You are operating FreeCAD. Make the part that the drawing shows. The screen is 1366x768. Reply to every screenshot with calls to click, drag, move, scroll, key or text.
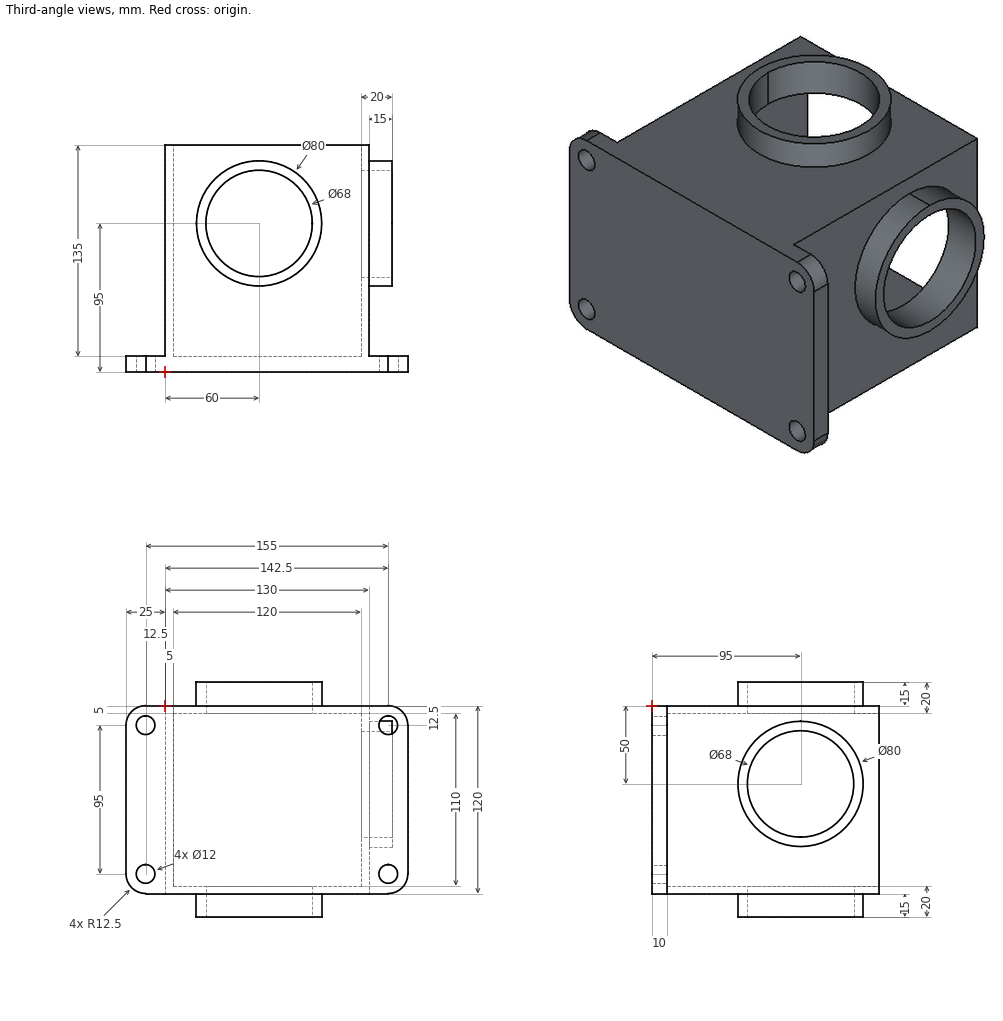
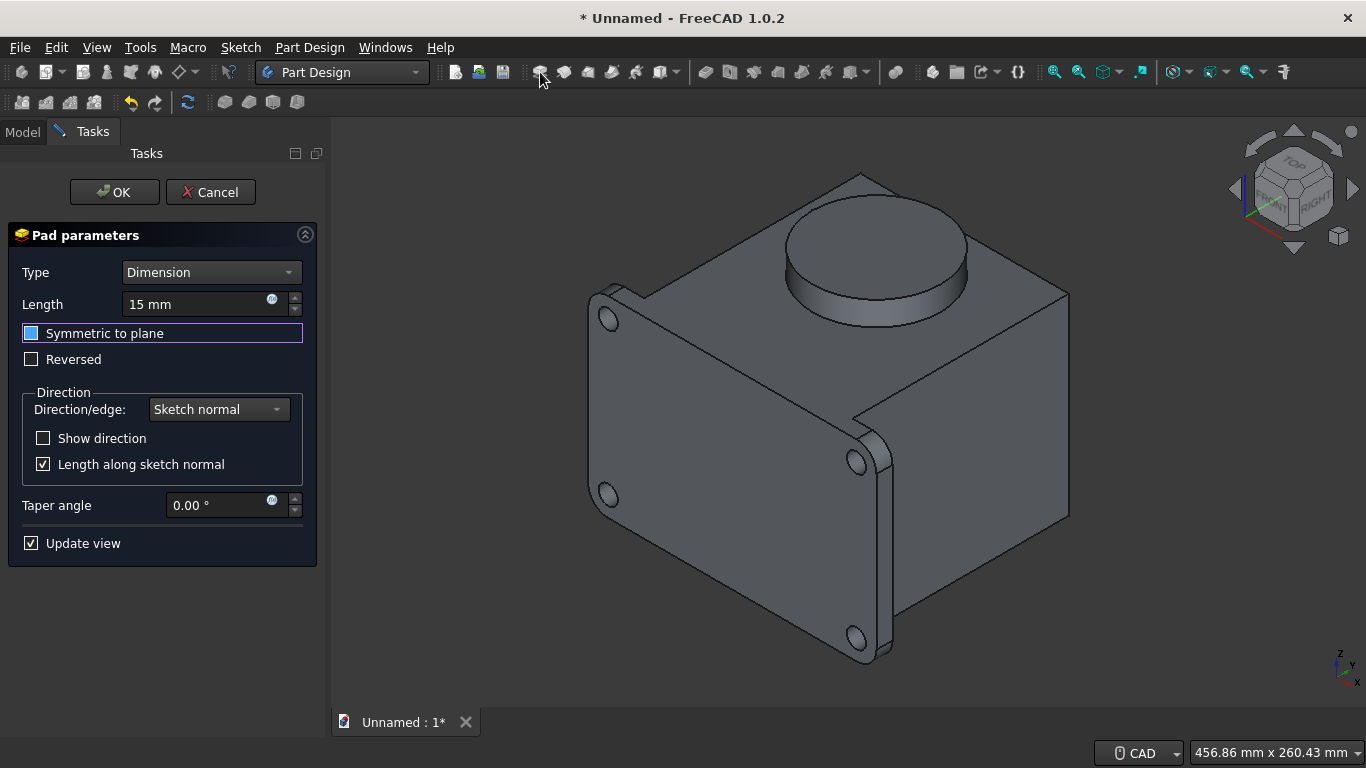
click(115, 192)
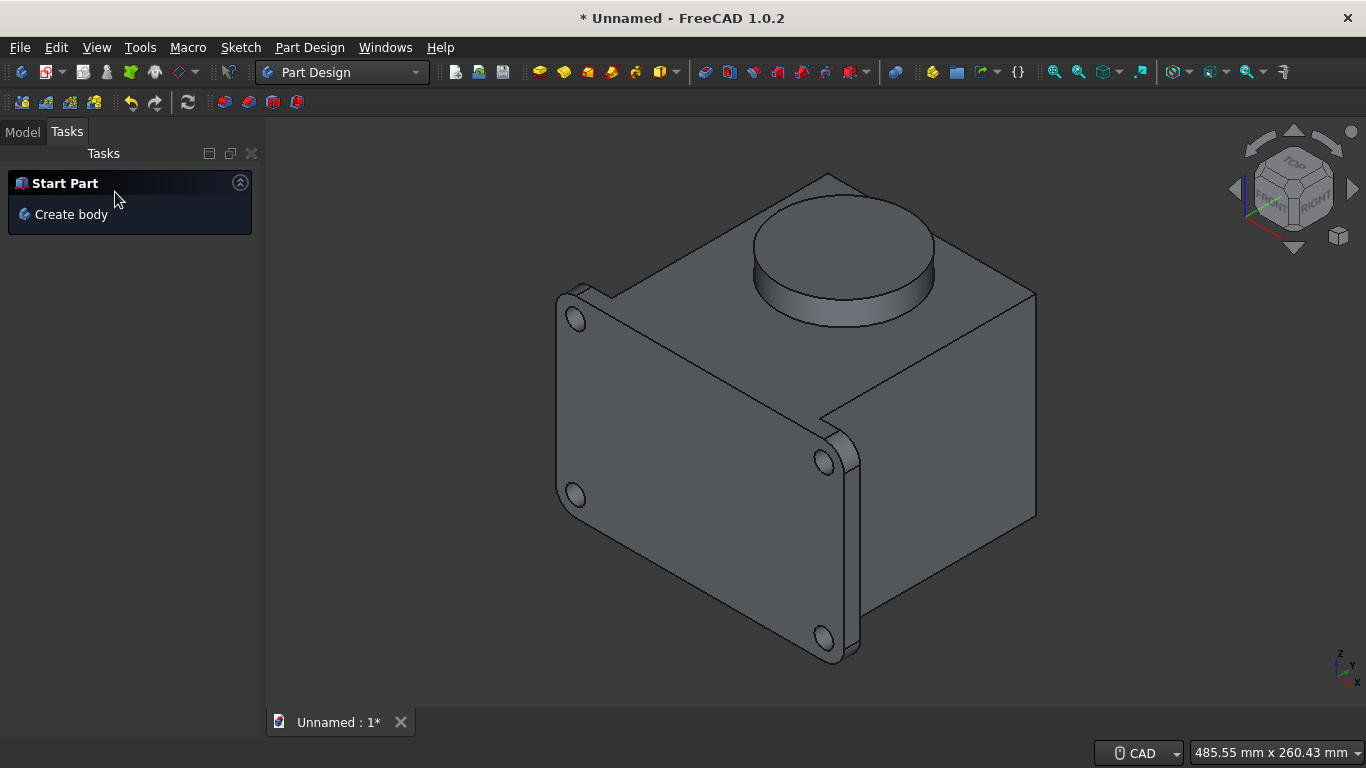
click(844, 246)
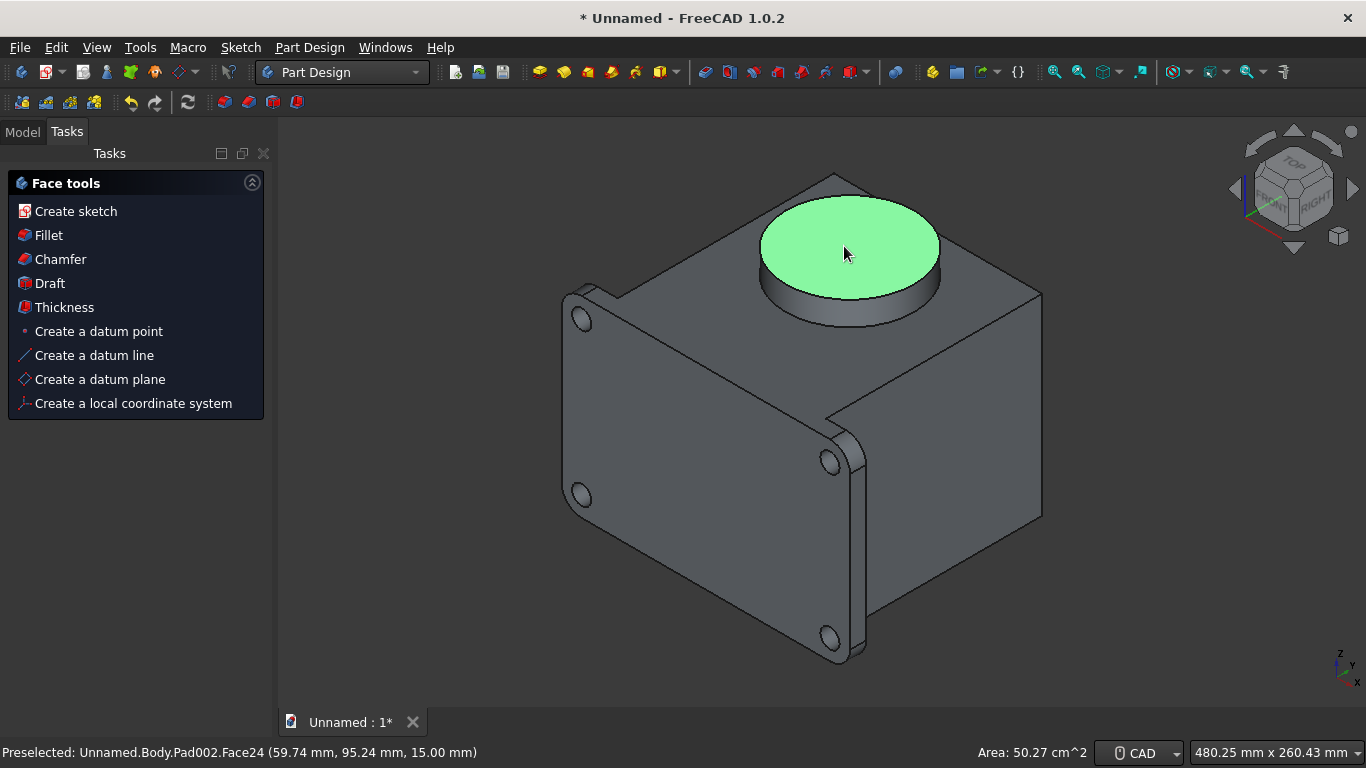
click(46, 72)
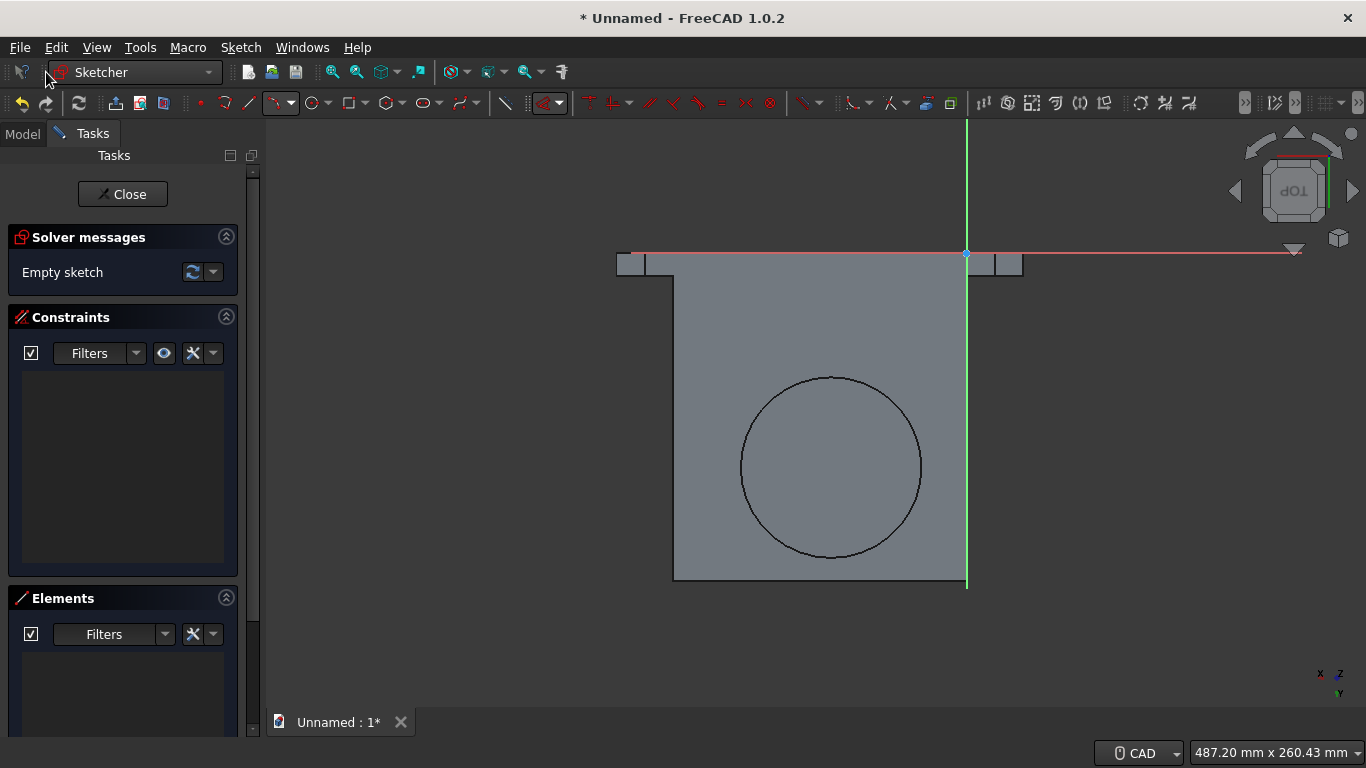
click(312, 104)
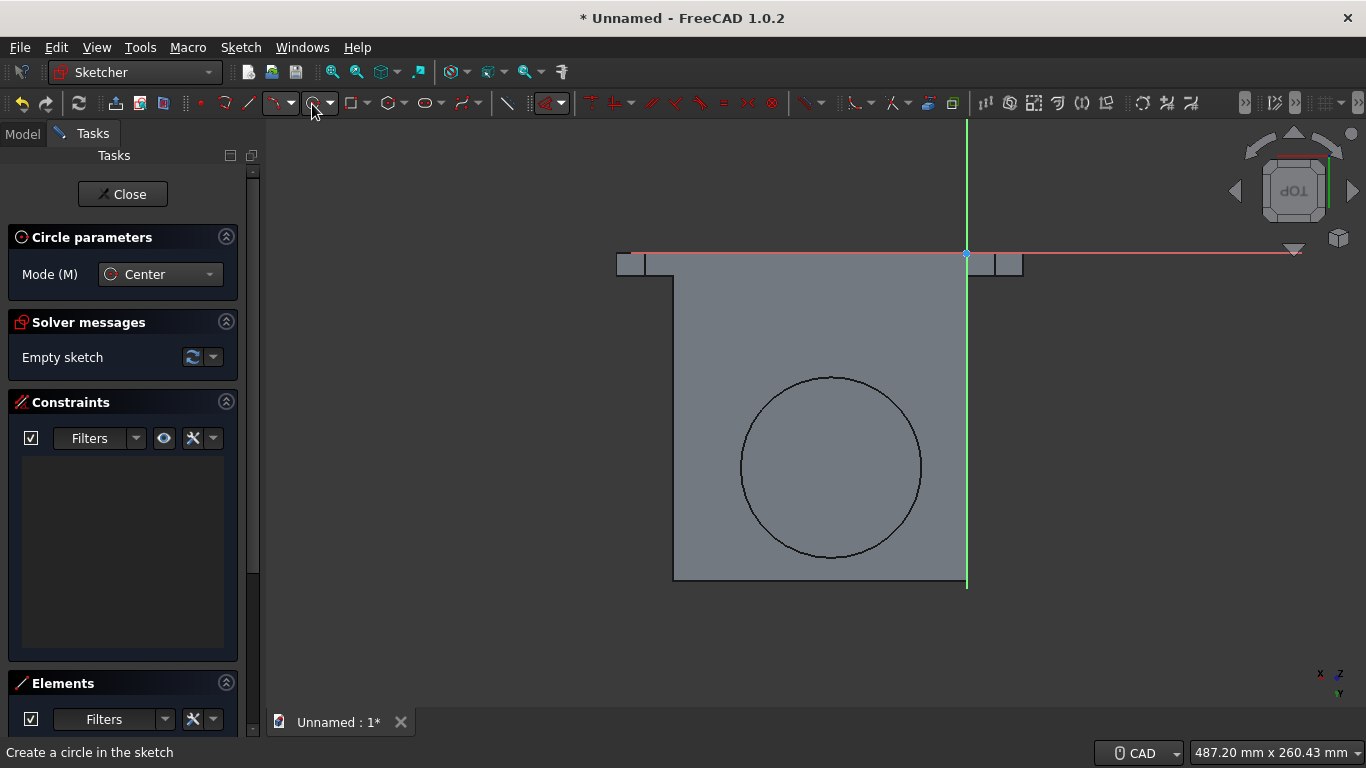
click(831, 468)
move(885, 413)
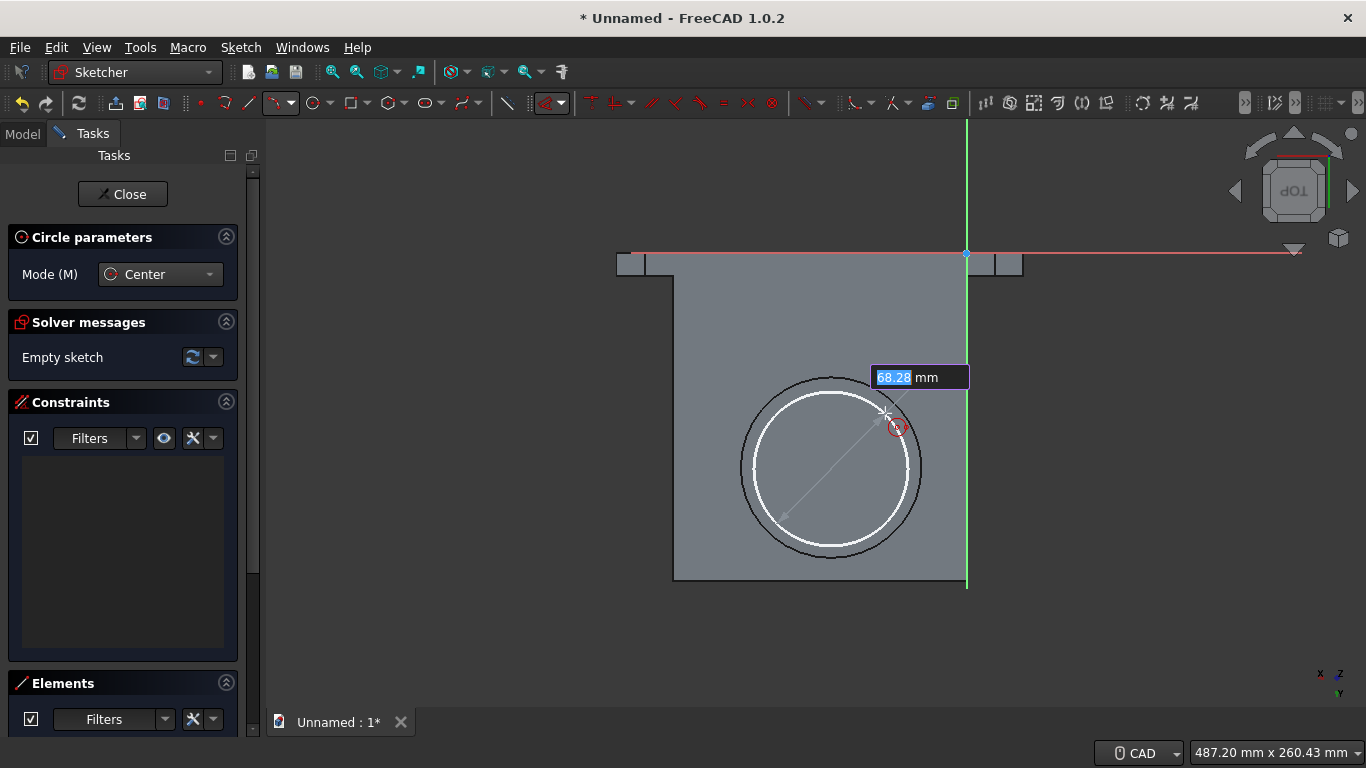
text(68)
key(Return)
key(Escape)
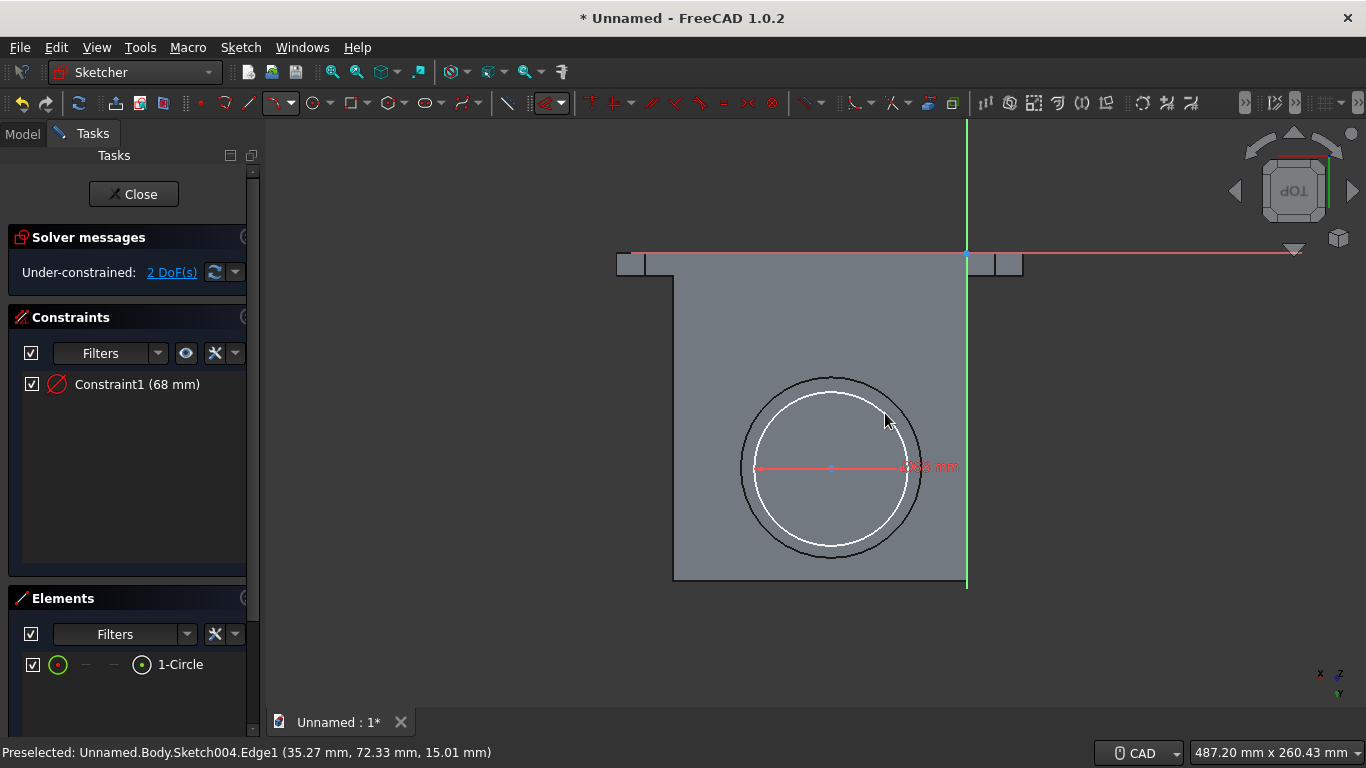
click(831, 469)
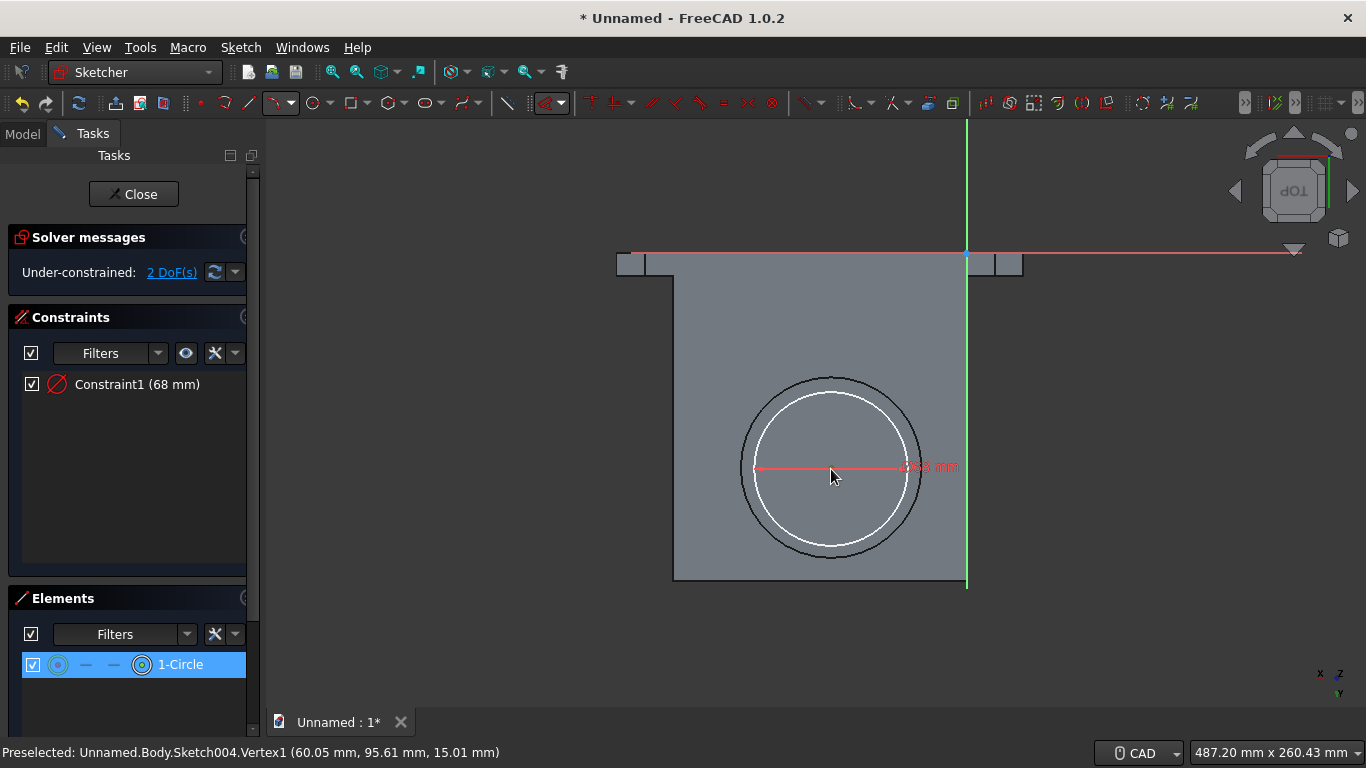
key(l)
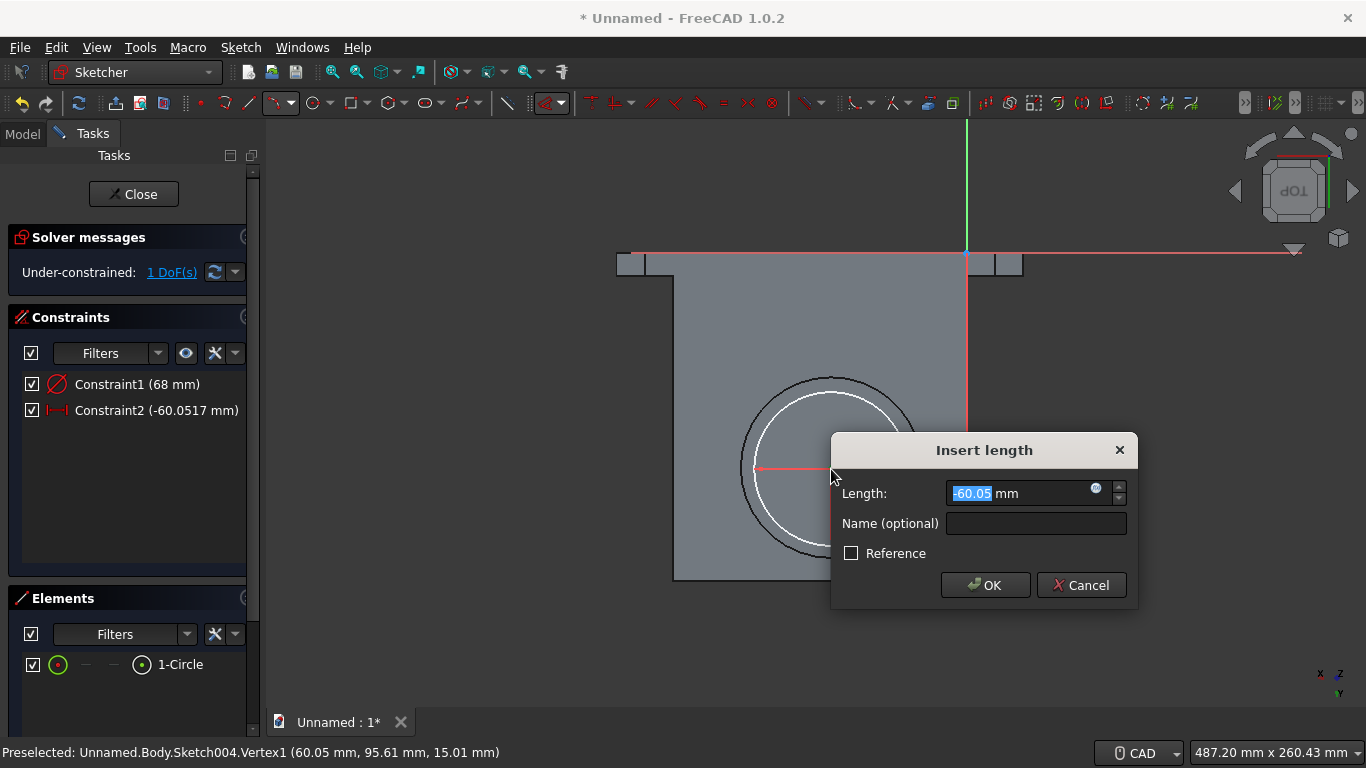
text(-60)
key(Return)